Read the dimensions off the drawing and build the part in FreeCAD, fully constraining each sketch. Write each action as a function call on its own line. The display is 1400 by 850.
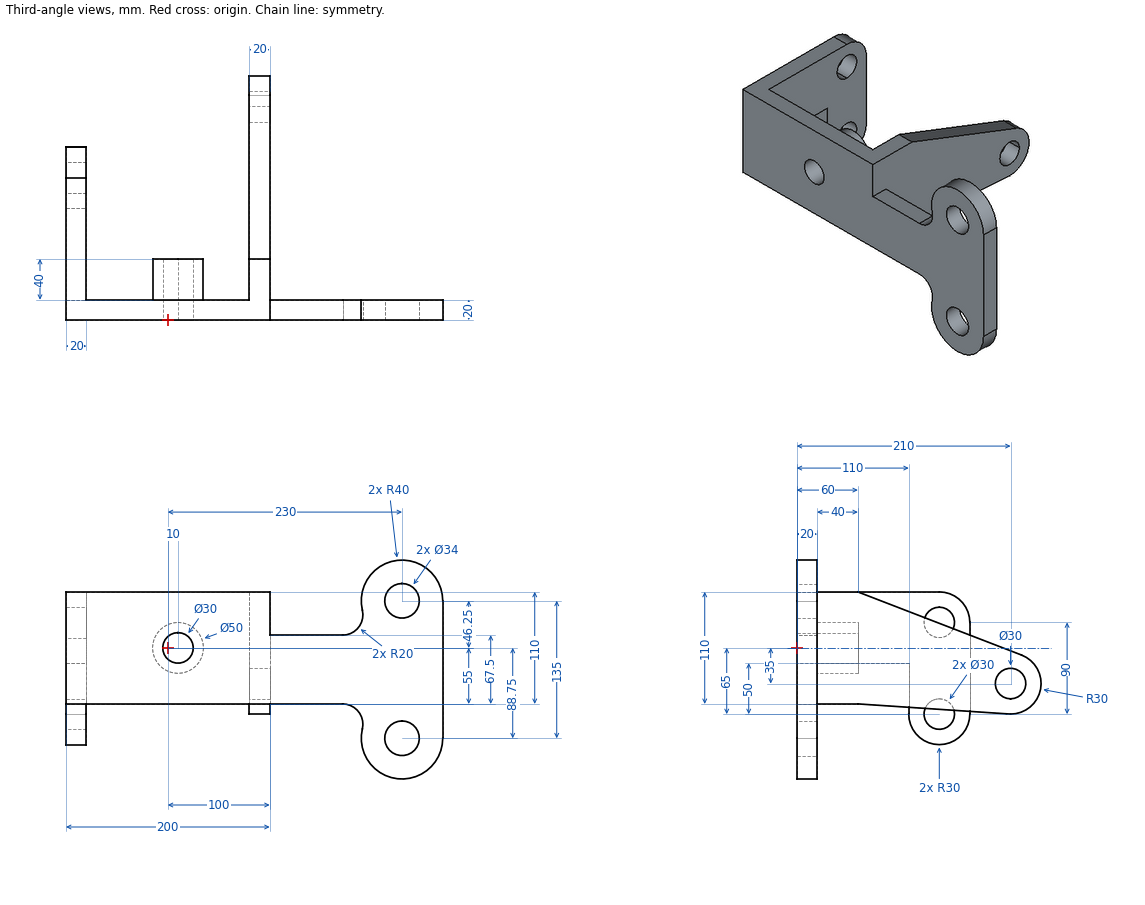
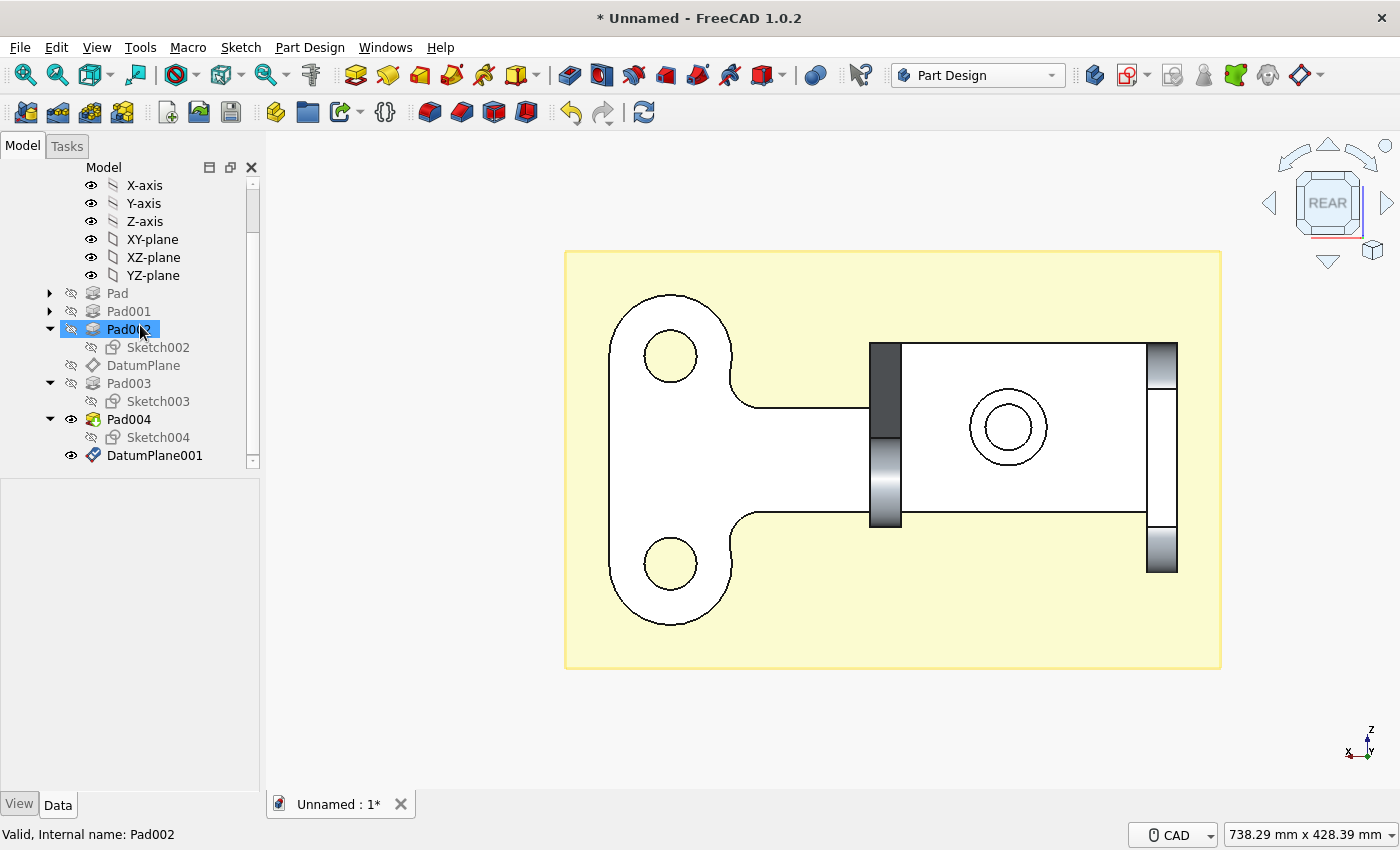
click(116, 455)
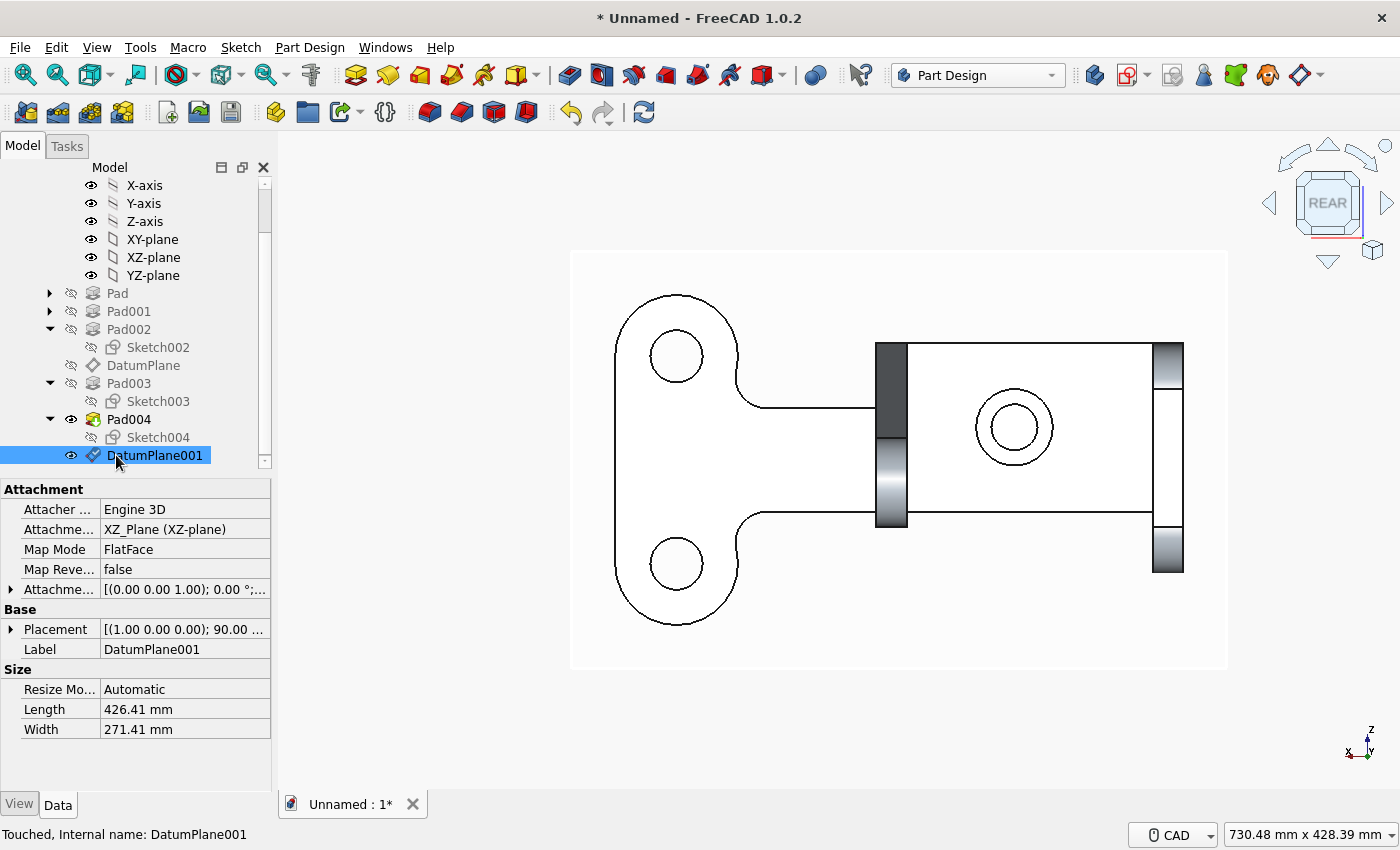
click(1128, 76)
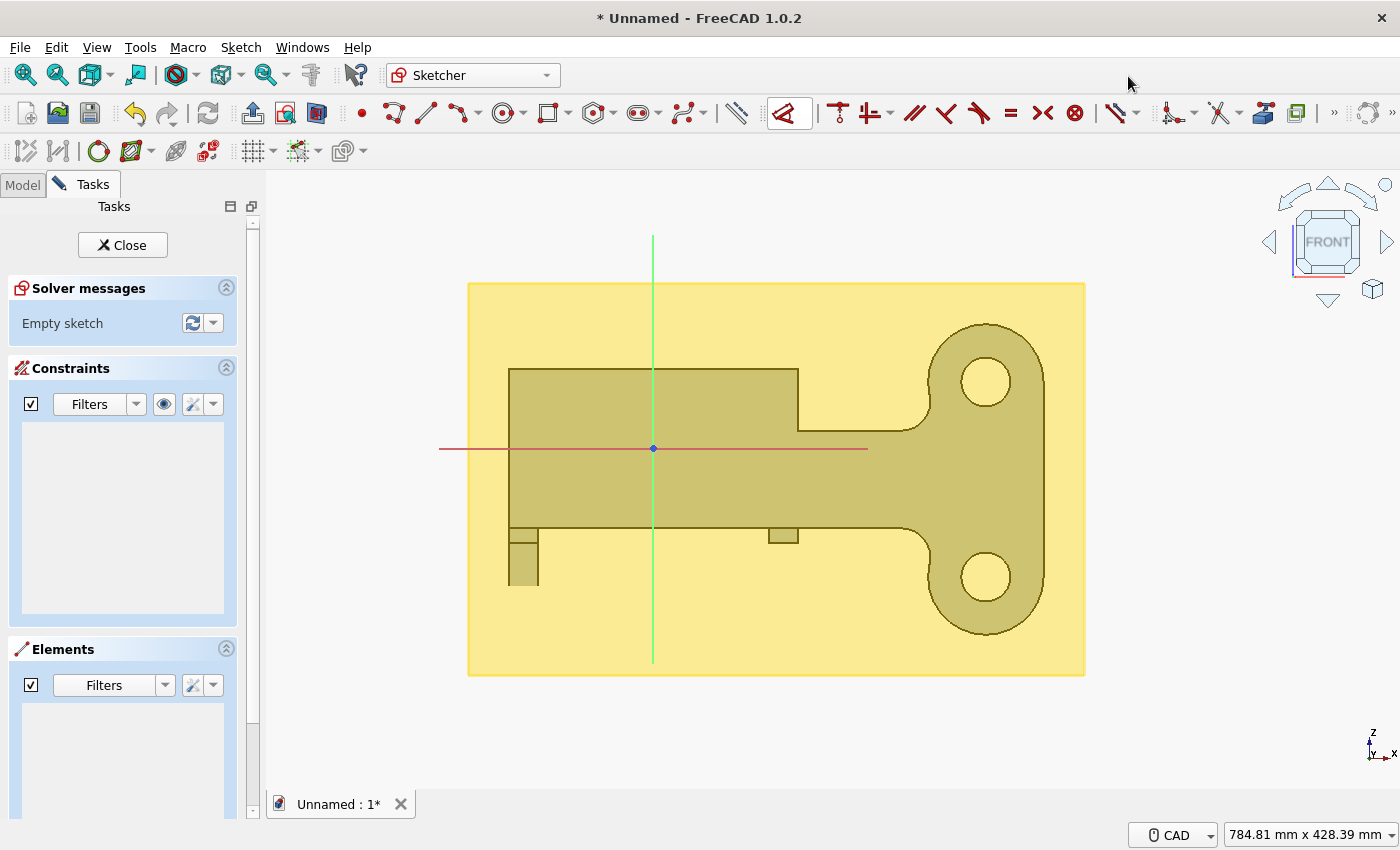
scroll(656, 445, up, 11)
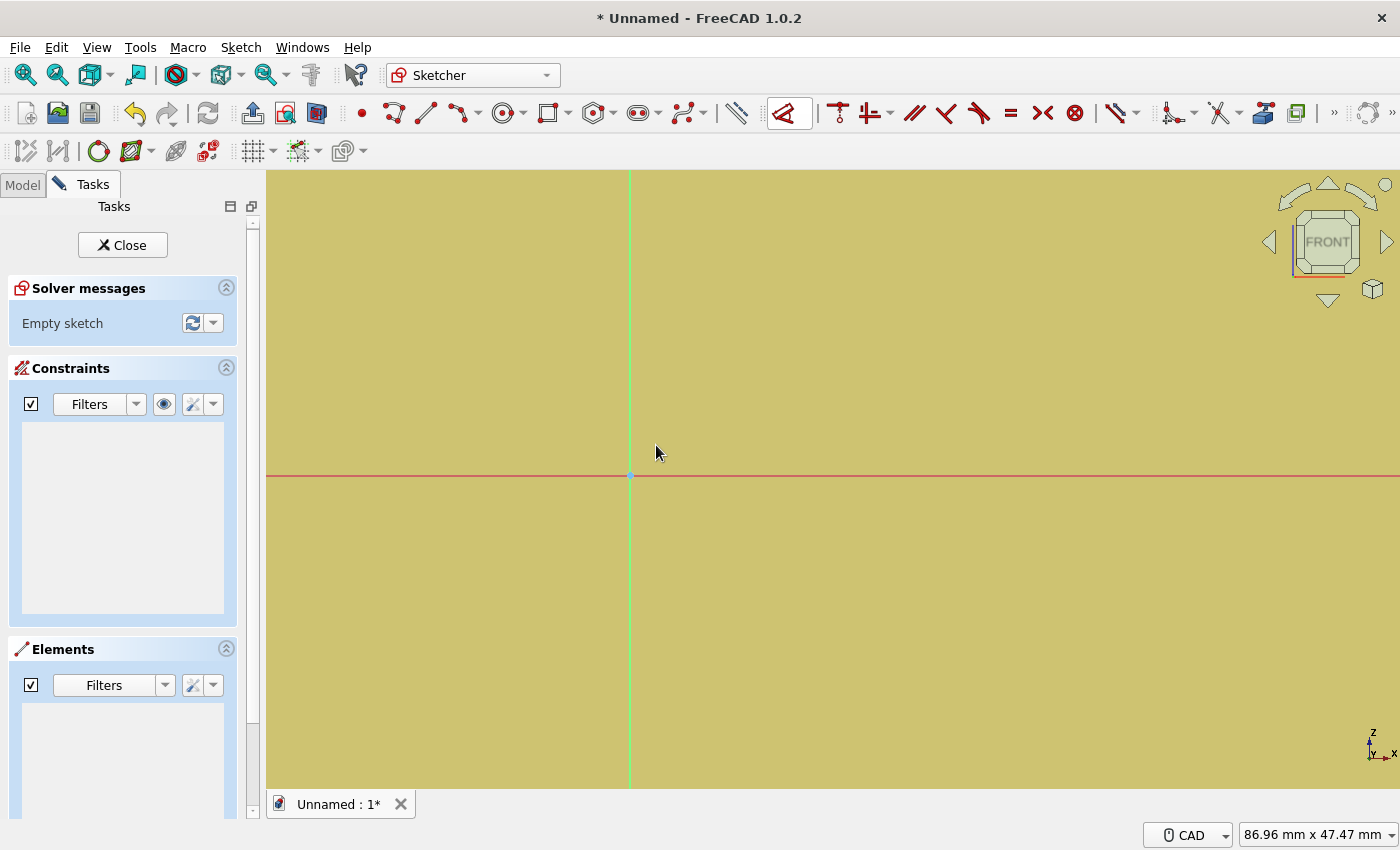
key(g)
key(c)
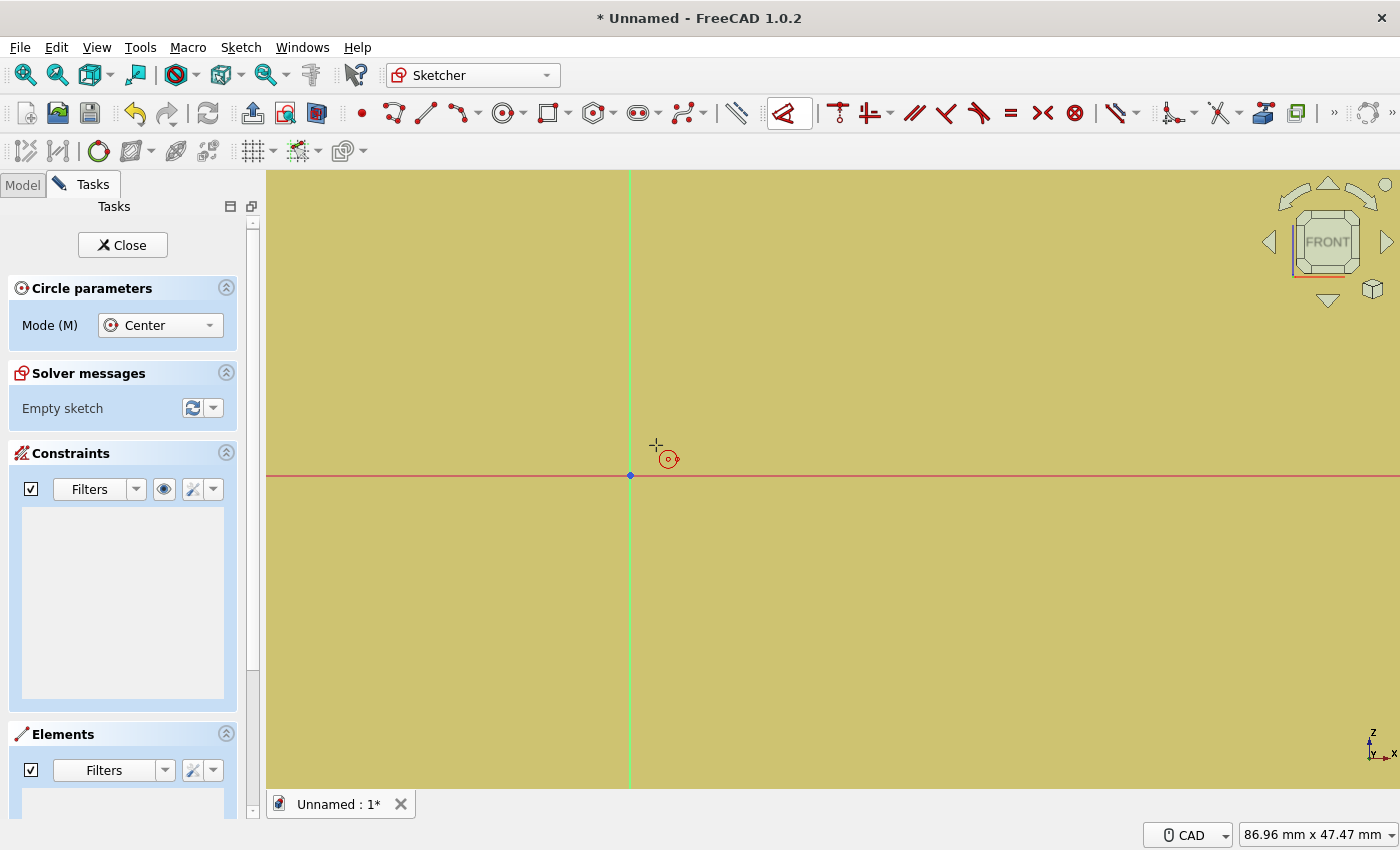
click(761, 476)
click(899, 337)
key(Escape)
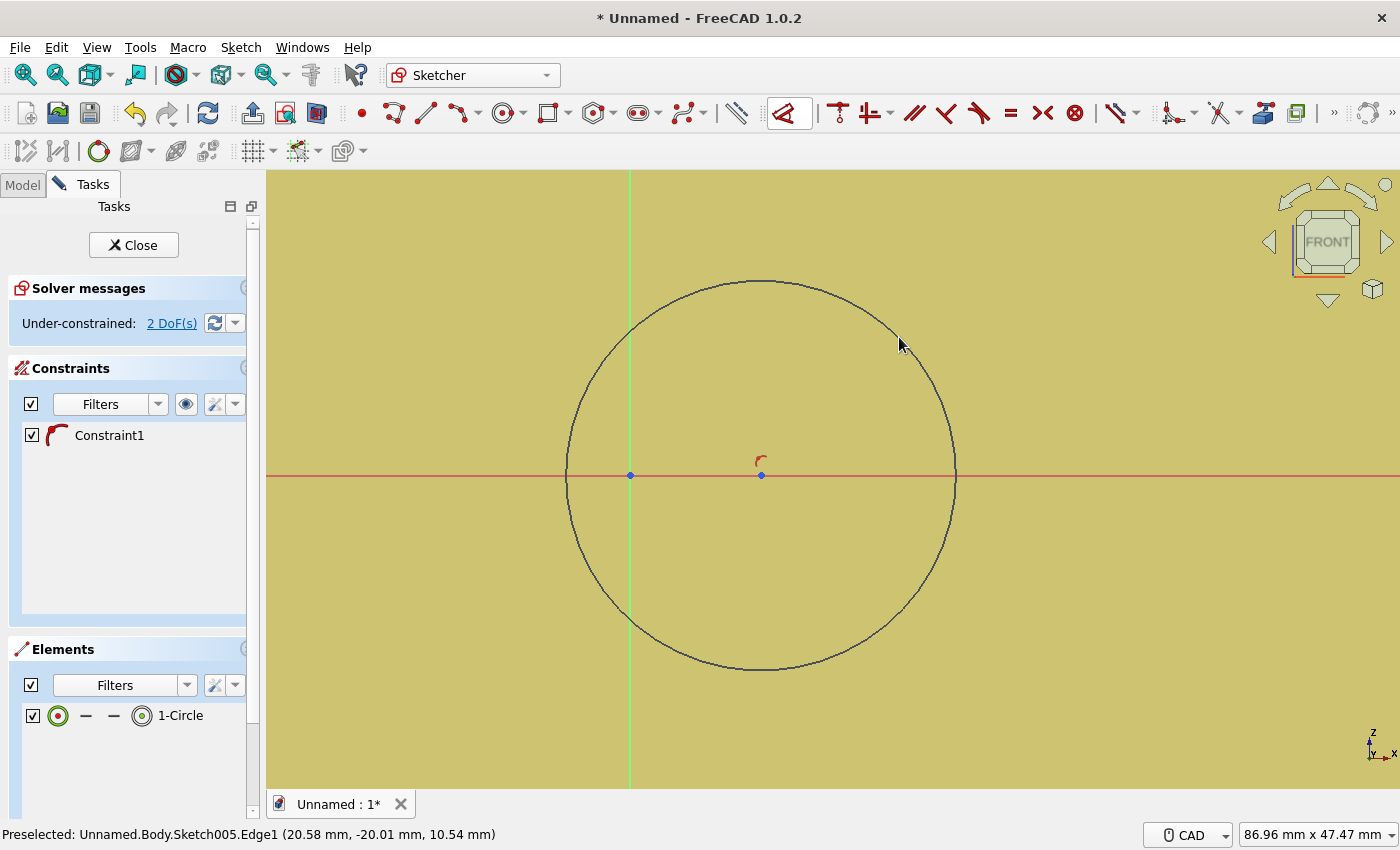
click(898, 337)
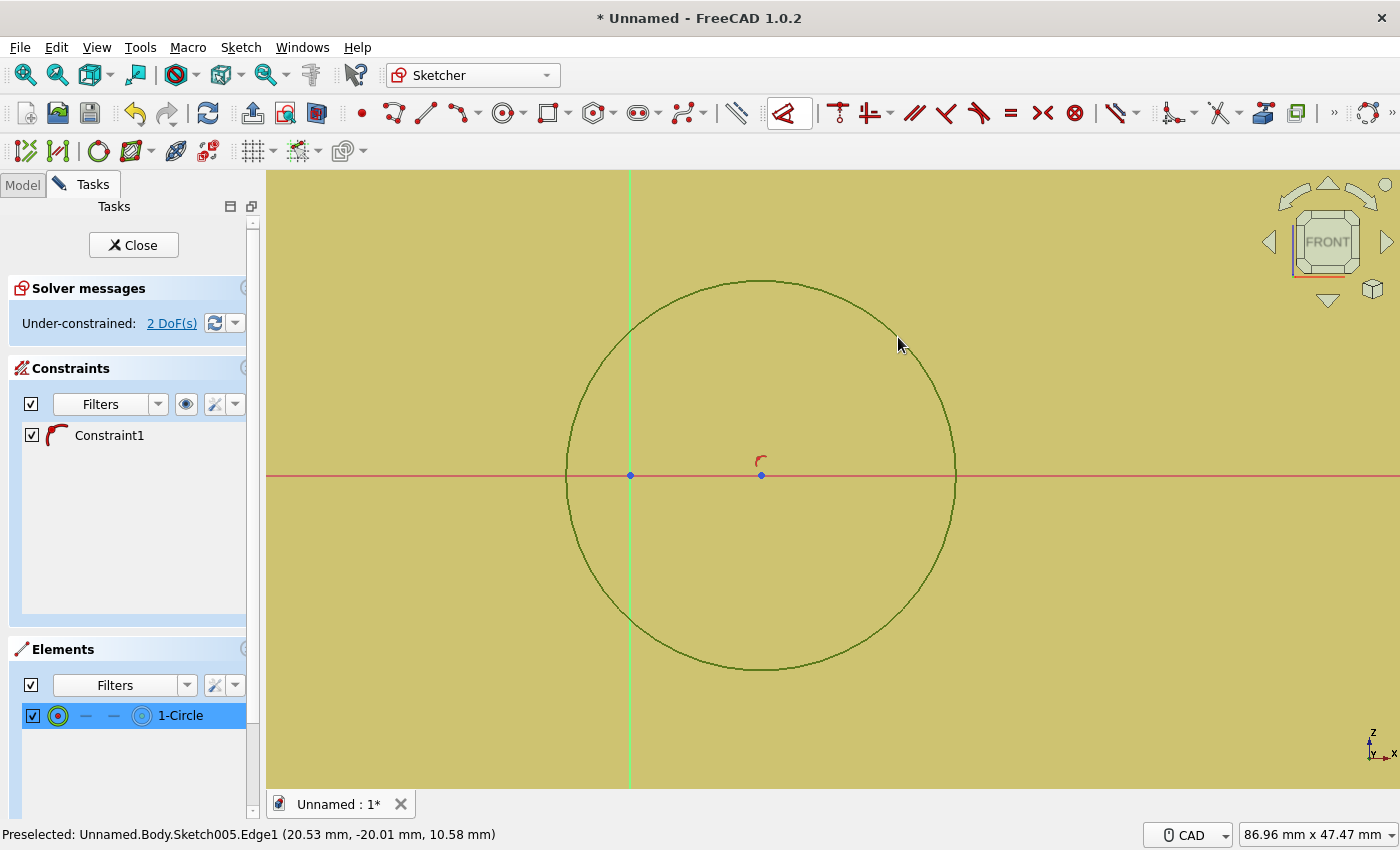
key(k)
key(o)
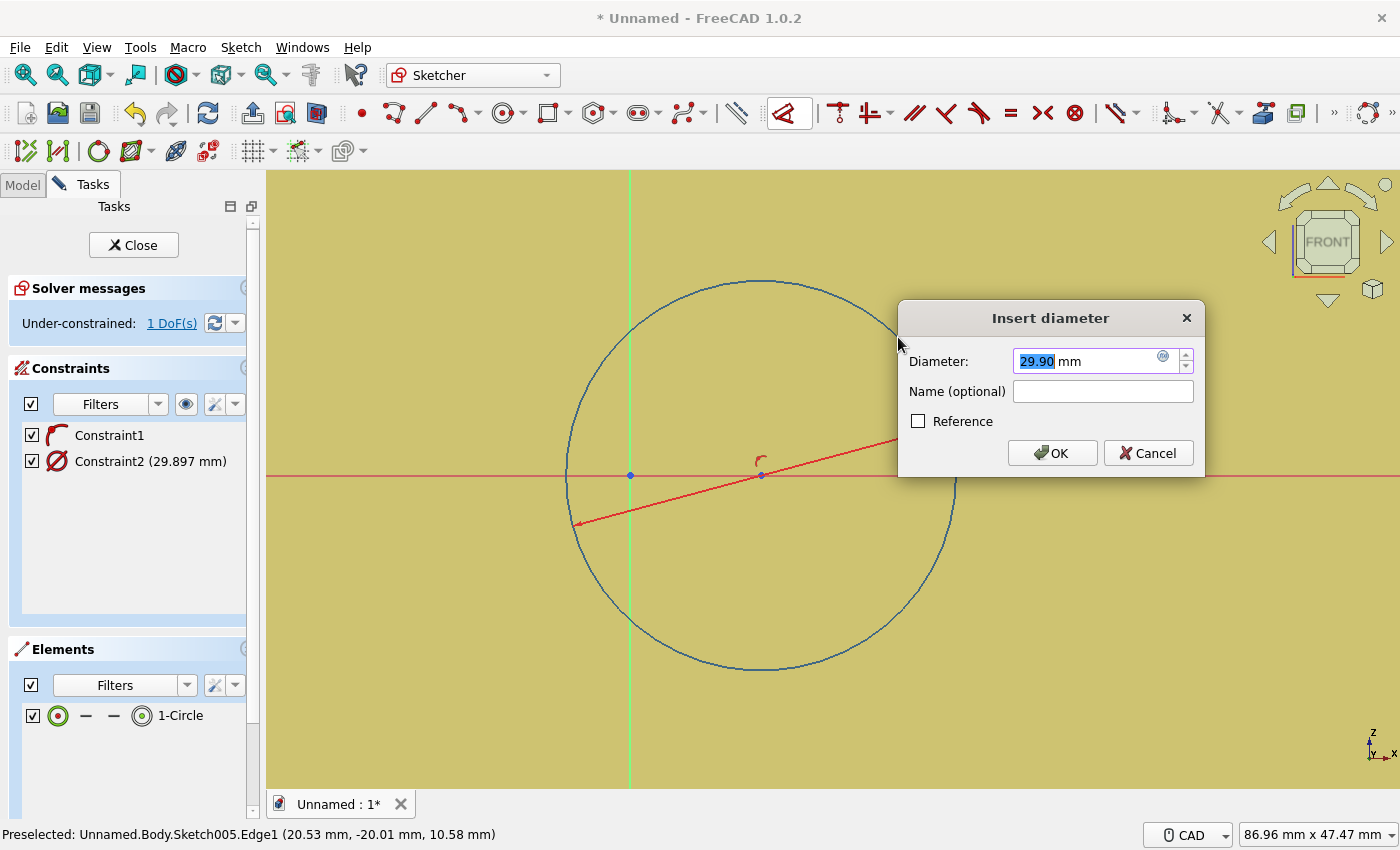
text(30)
key(Return)